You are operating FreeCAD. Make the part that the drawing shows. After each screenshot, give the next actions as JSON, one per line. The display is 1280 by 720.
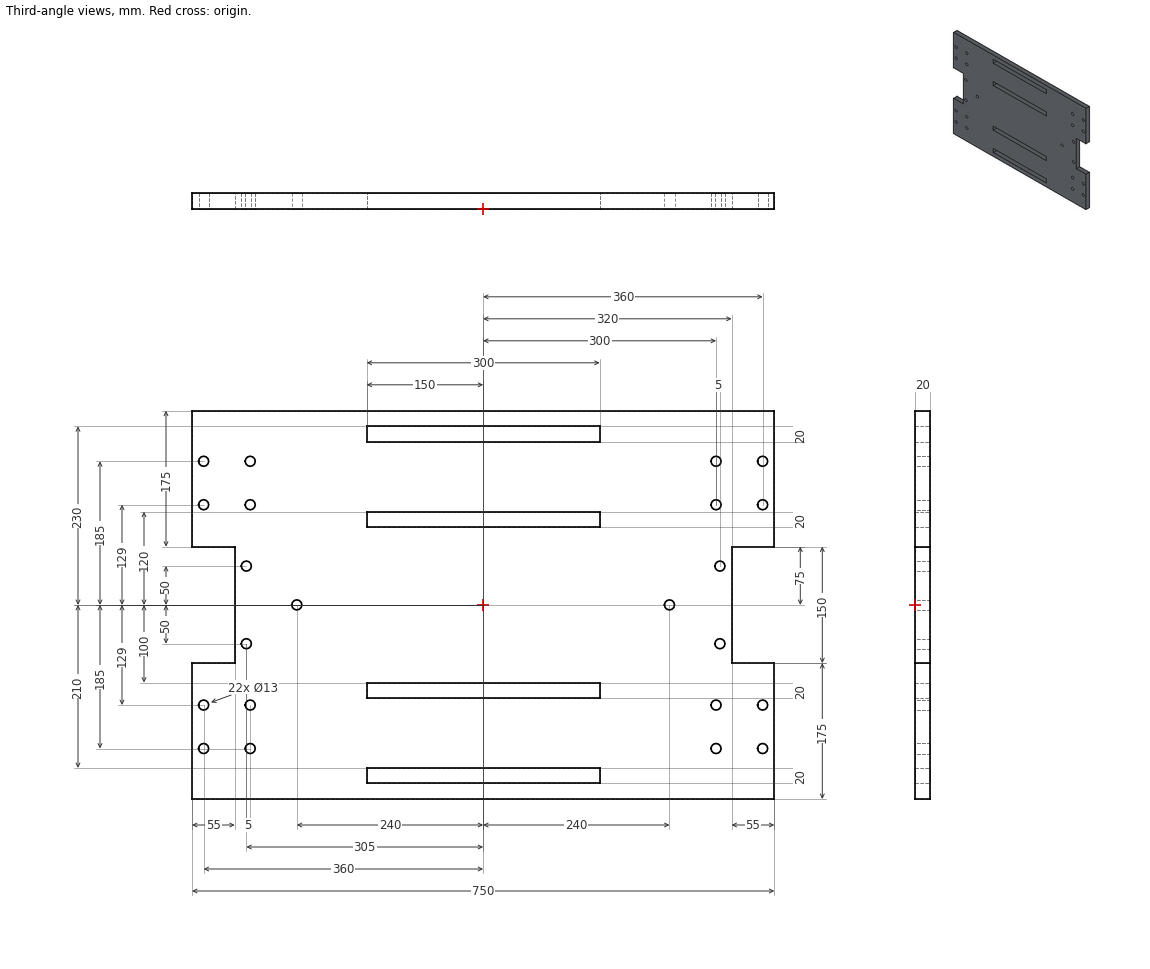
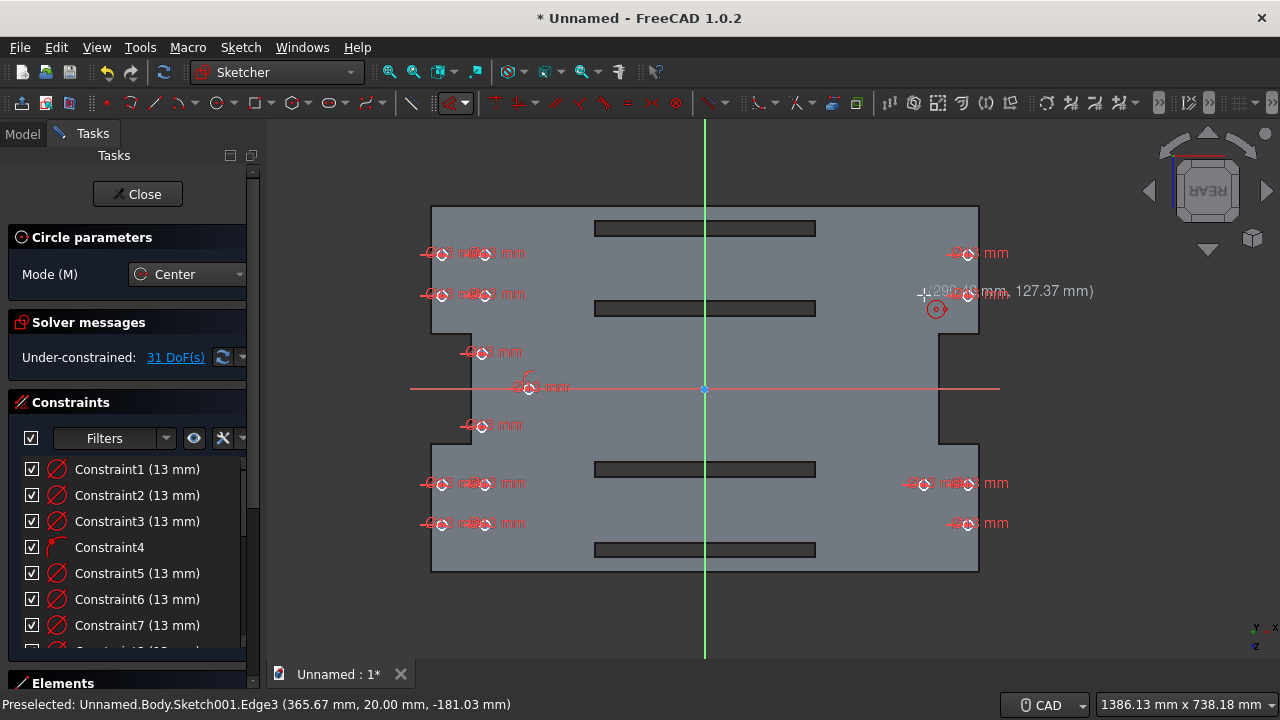
{"action": "left_click", "coordinate": [924, 295]}
{"action": "mouse_move", "coordinate": [928, 291]}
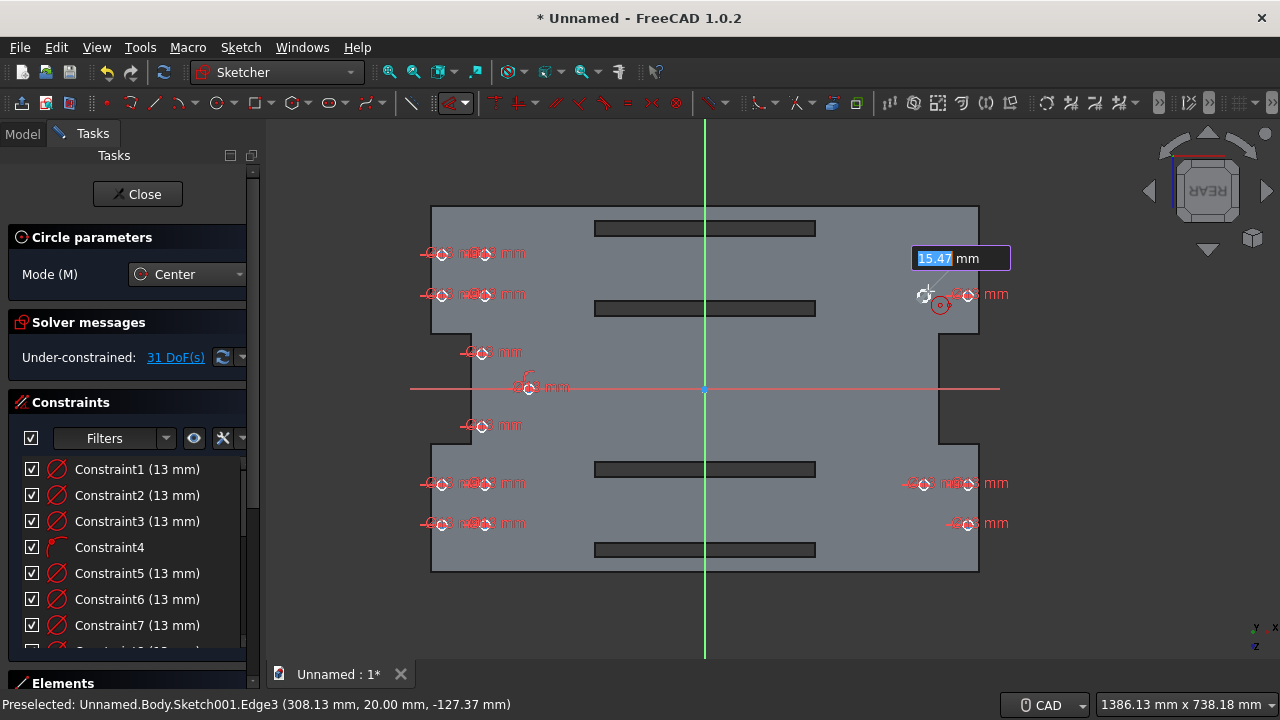
{"action": "type", "text": "13"}
{"action": "key", "text": "Return"}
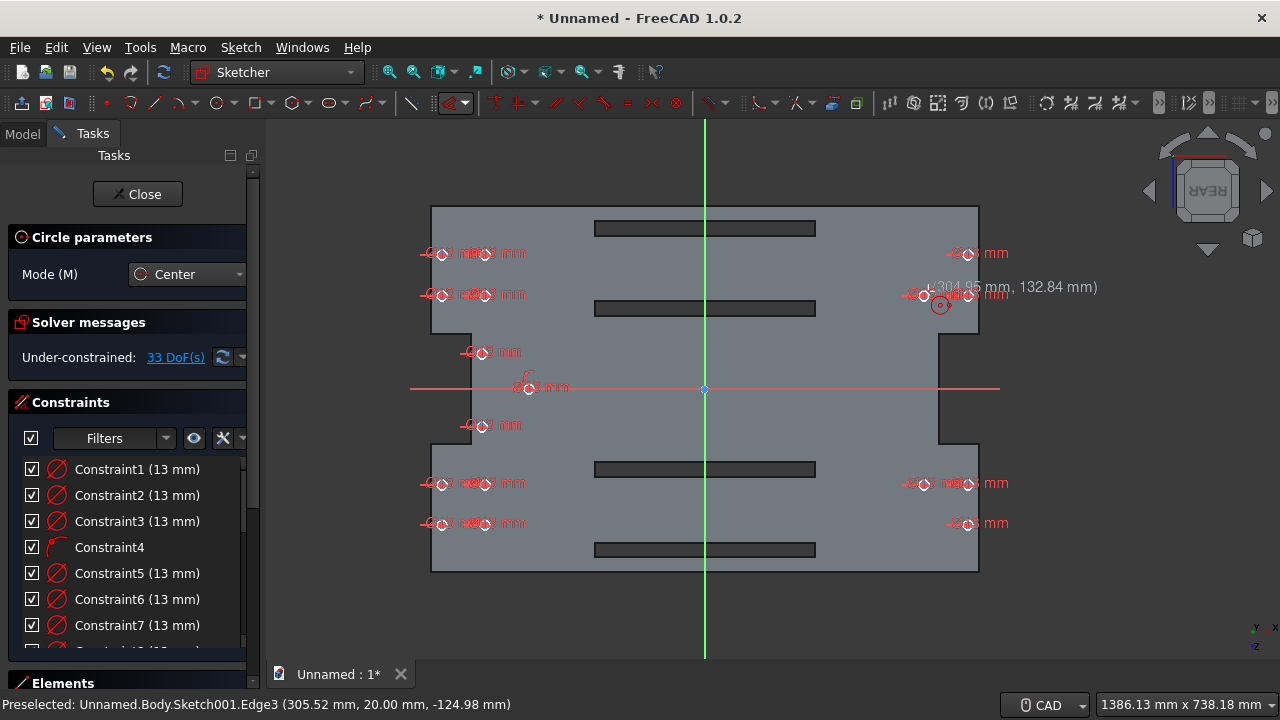
{"action": "scroll", "coordinate": [928, 426], "scroll_direction": "up", "scroll_amount": 8}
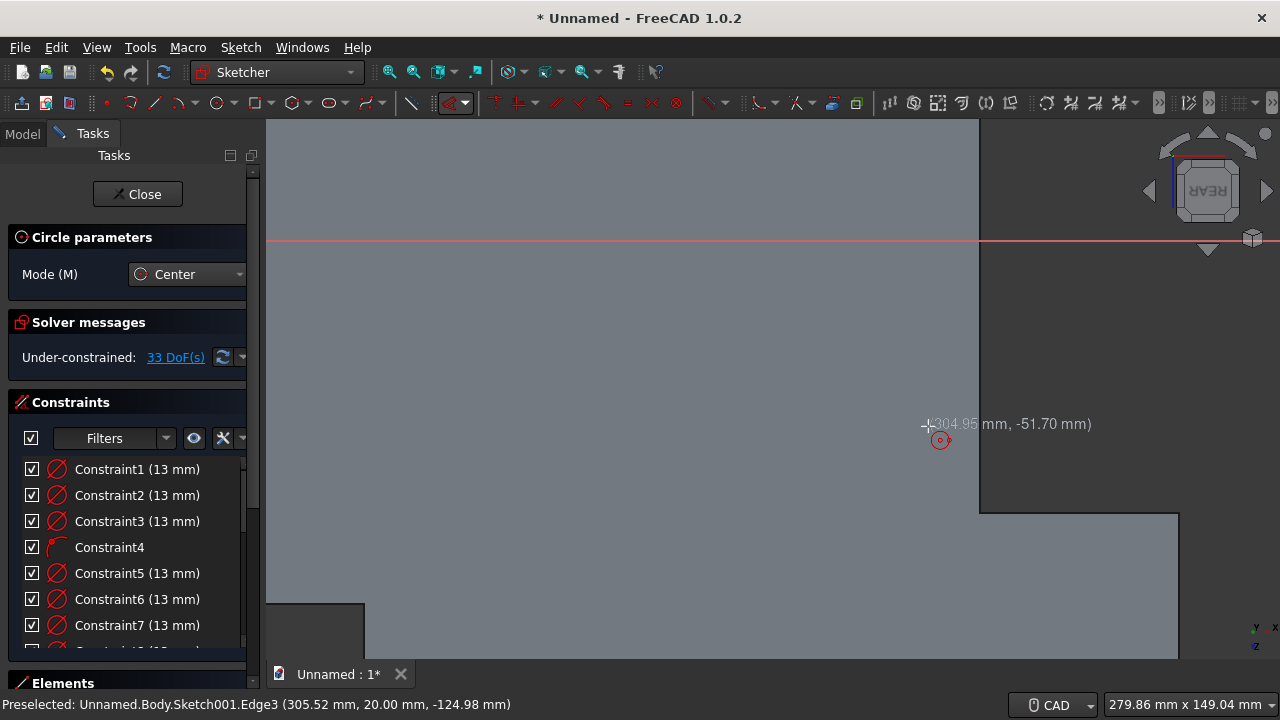
{"action": "scroll", "coordinate": [928, 426], "scroll_direction": "down", "scroll_amount": 8}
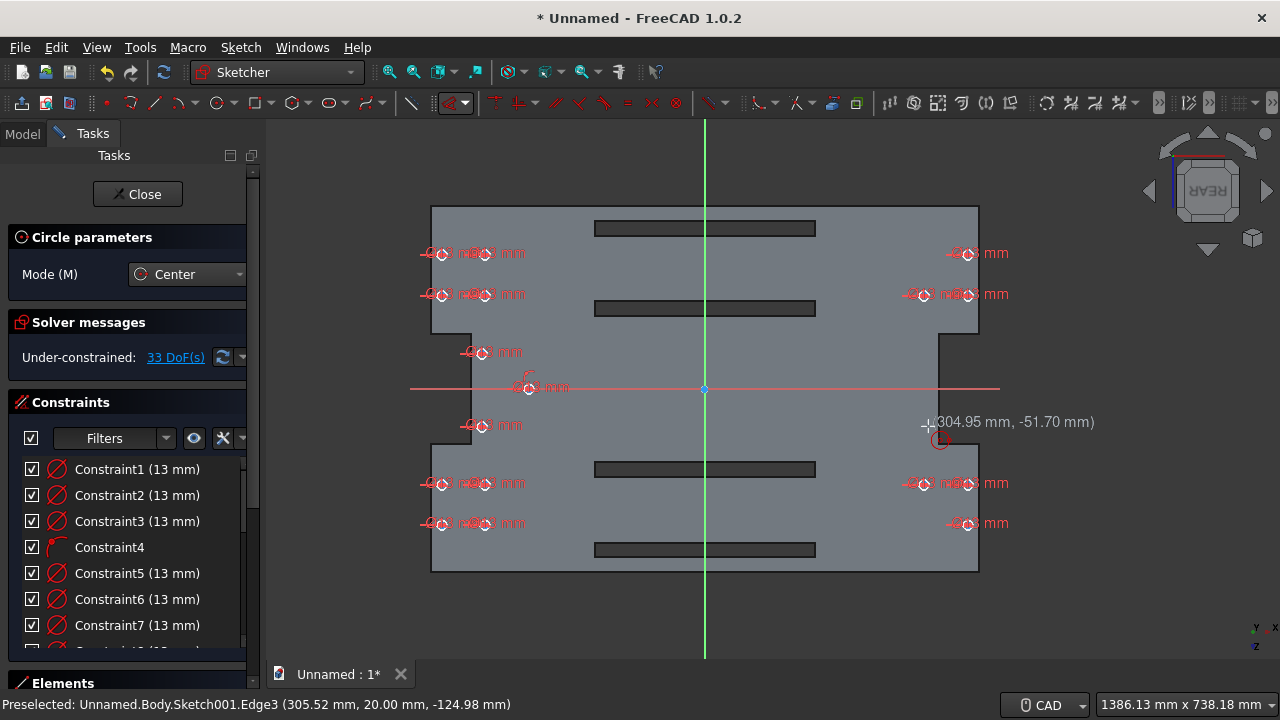
{"action": "left_click", "coordinate": [928, 426]}
{"action": "mouse_move", "coordinate": [931, 422]}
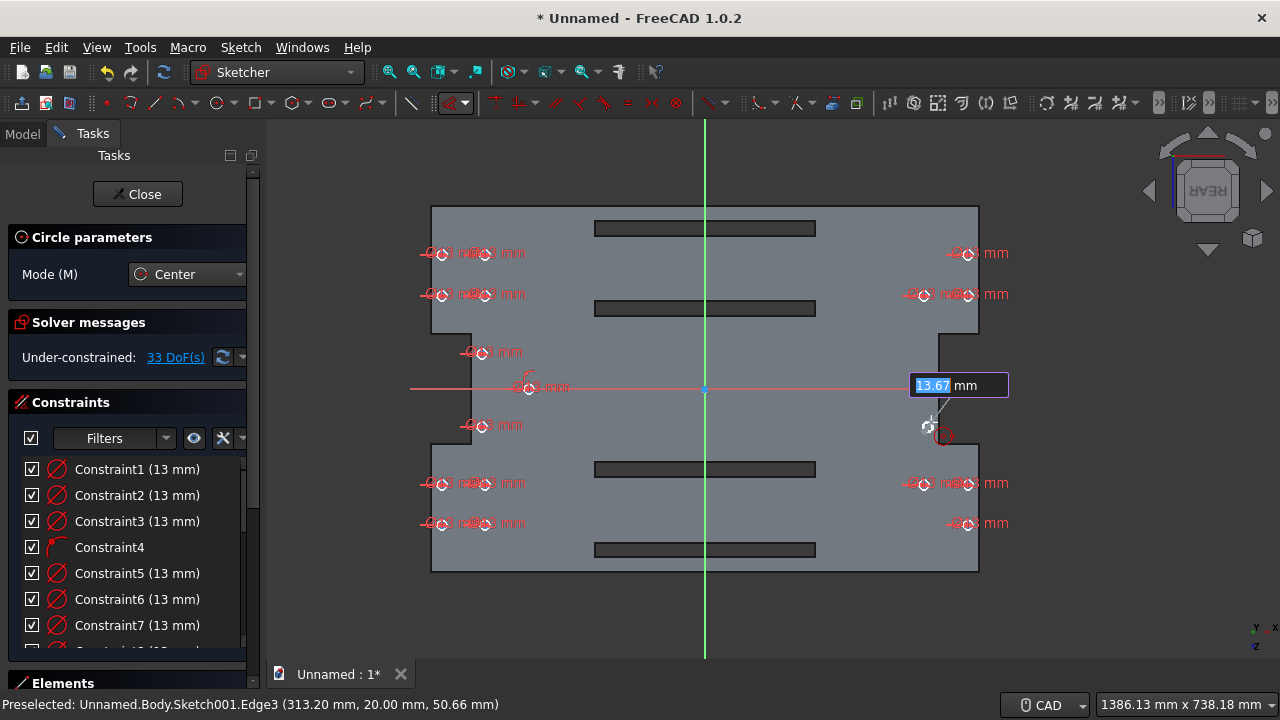
{"action": "type", "text": "13"}
{"action": "key", "text": "Return"}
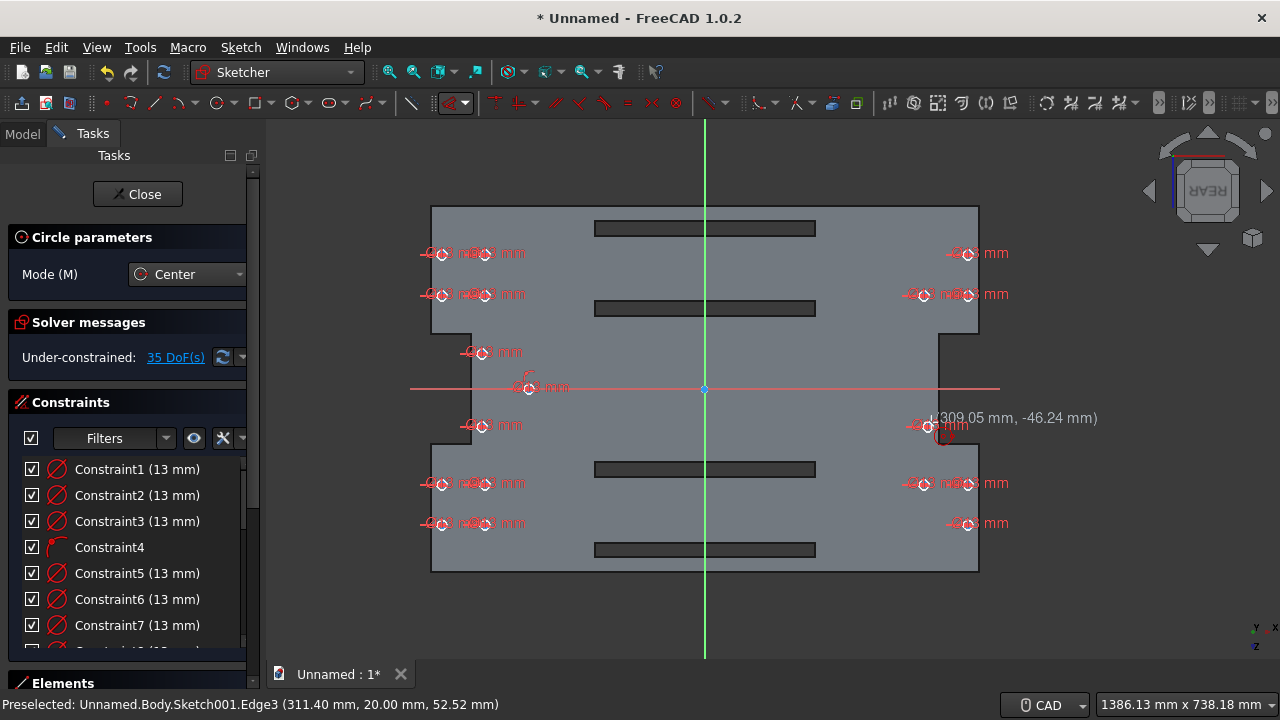
{"action": "scroll", "coordinate": [924, 525], "scroll_direction": "up", "scroll_amount": 8}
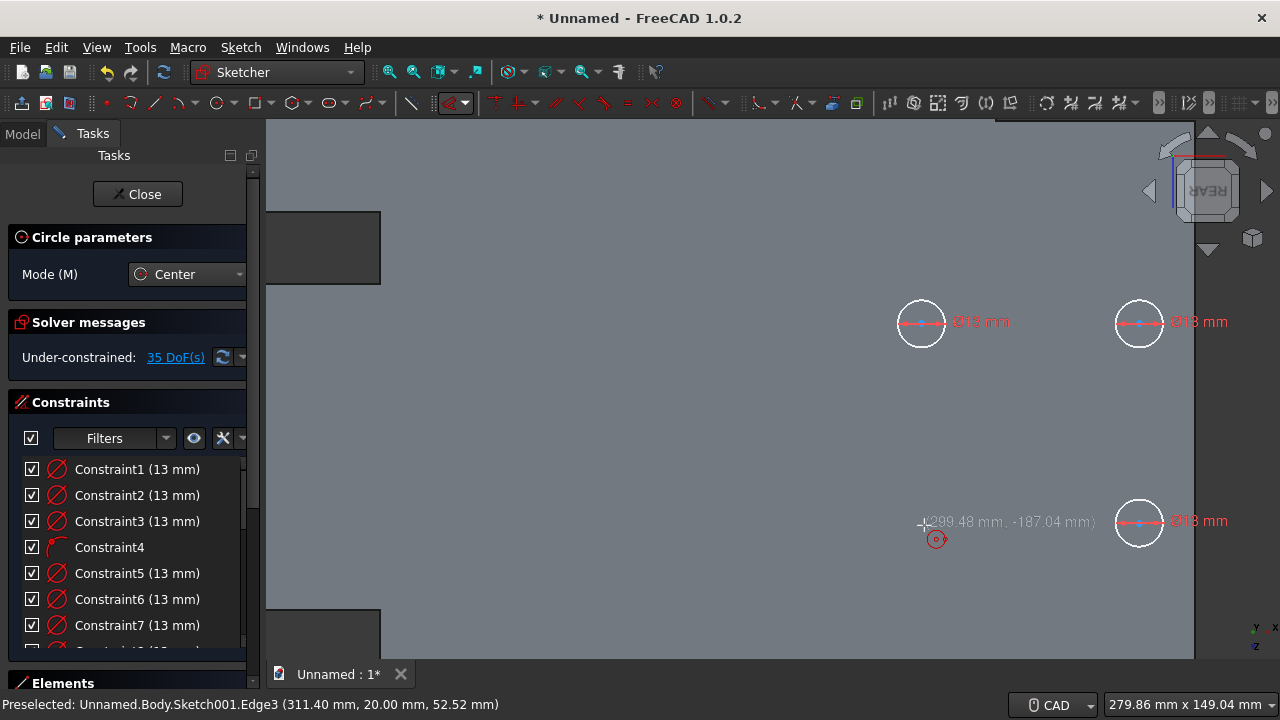
{"action": "scroll", "coordinate": [924, 526], "scroll_direction": "down", "scroll_amount": 8}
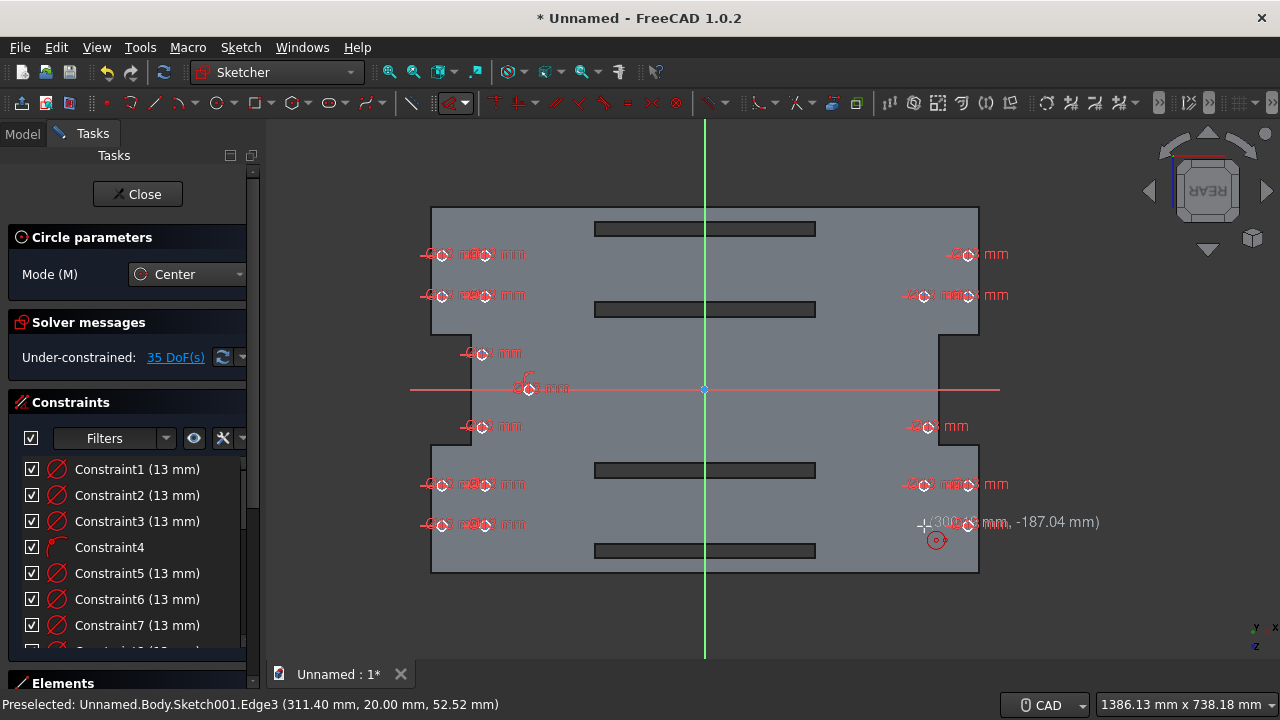
{"action": "left_click", "coordinate": [924, 525]}
{"action": "mouse_move", "coordinate": [928, 522]}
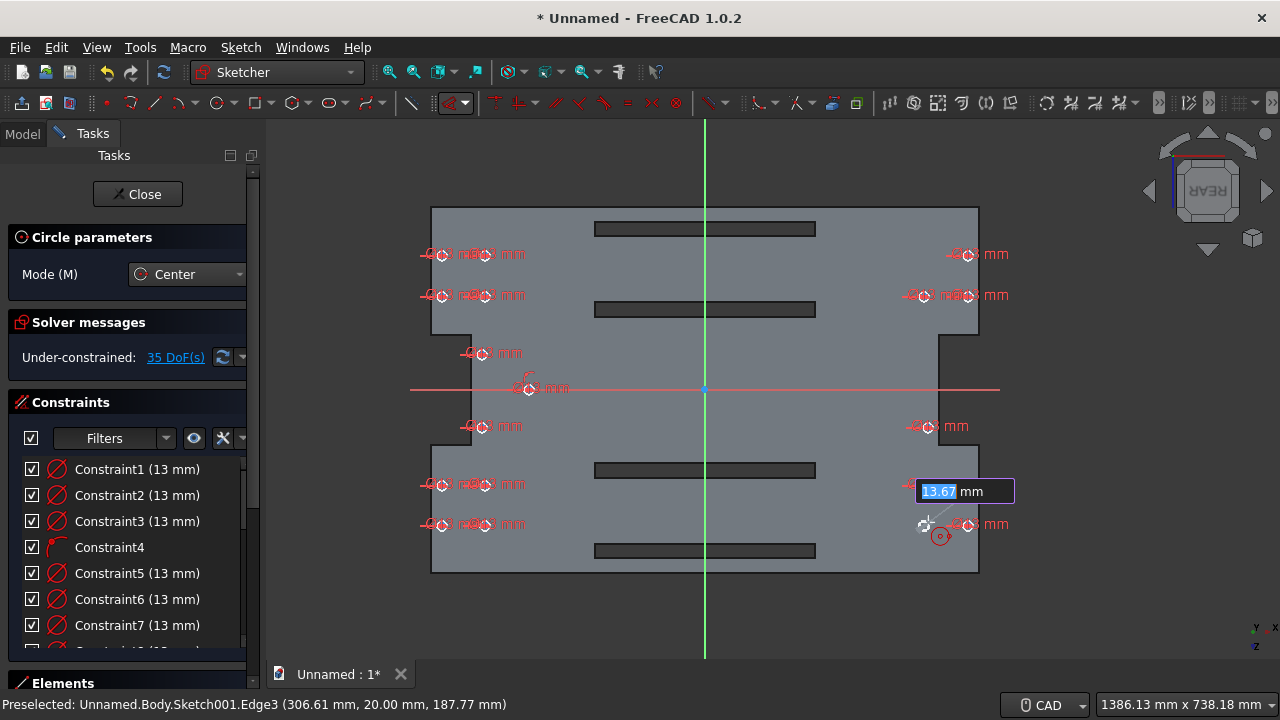
{"action": "type", "text": "13"}
{"action": "key", "text": "Return"}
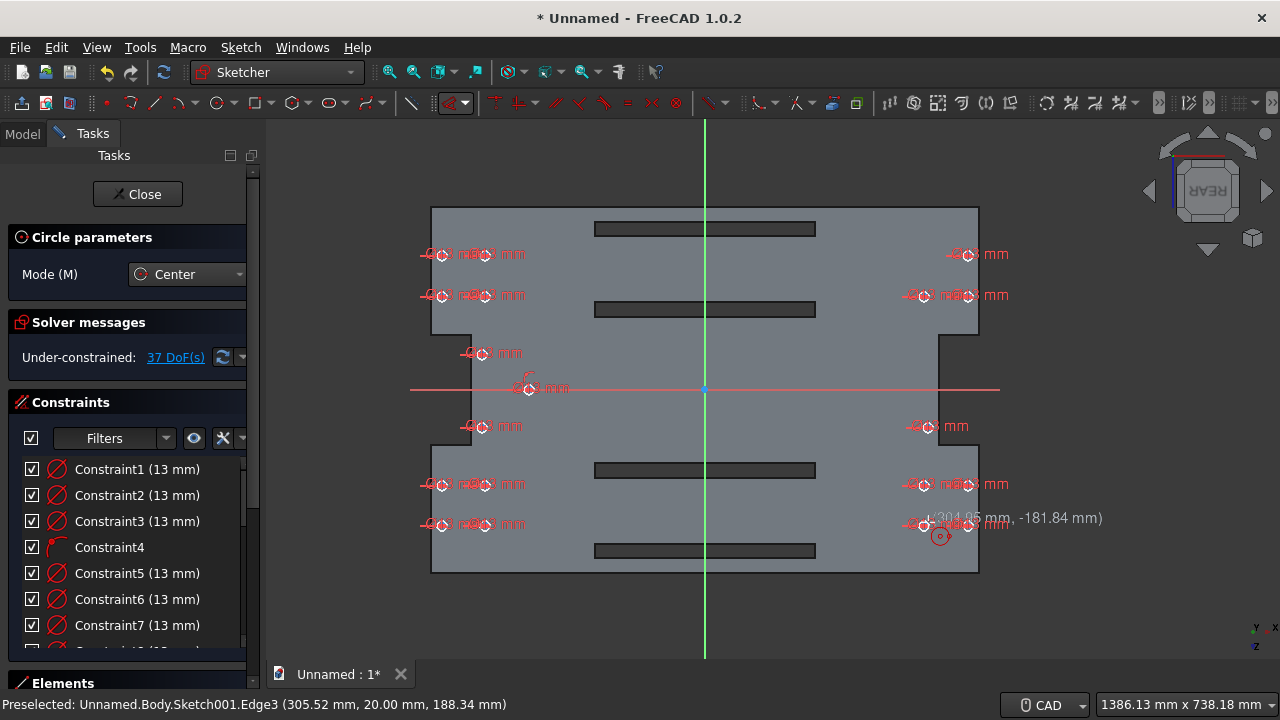
{"action": "scroll", "coordinate": [924, 255], "scroll_direction": "up", "scroll_amount": 8}